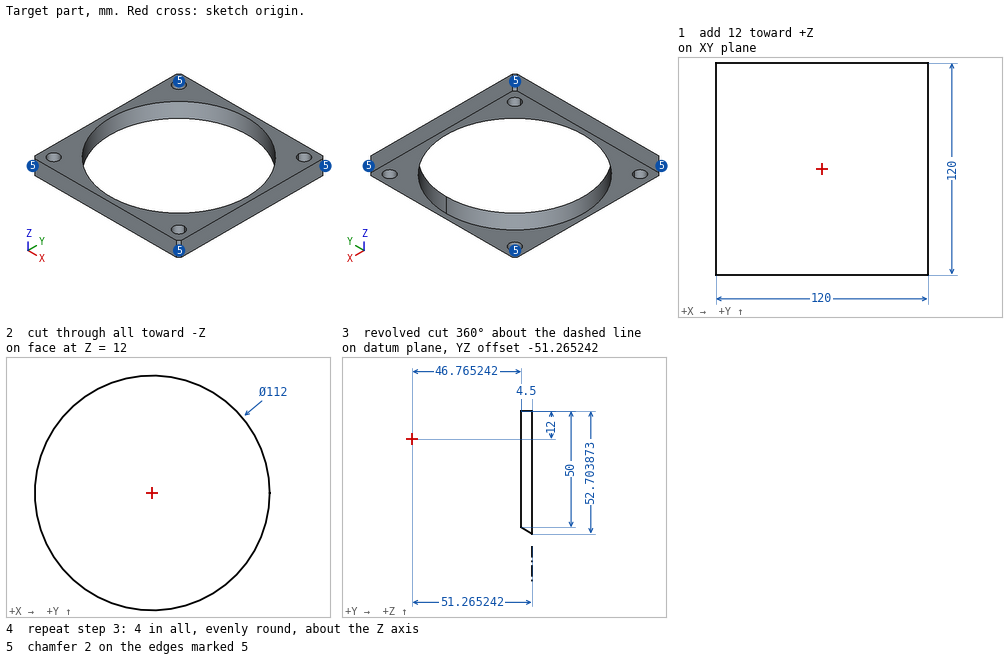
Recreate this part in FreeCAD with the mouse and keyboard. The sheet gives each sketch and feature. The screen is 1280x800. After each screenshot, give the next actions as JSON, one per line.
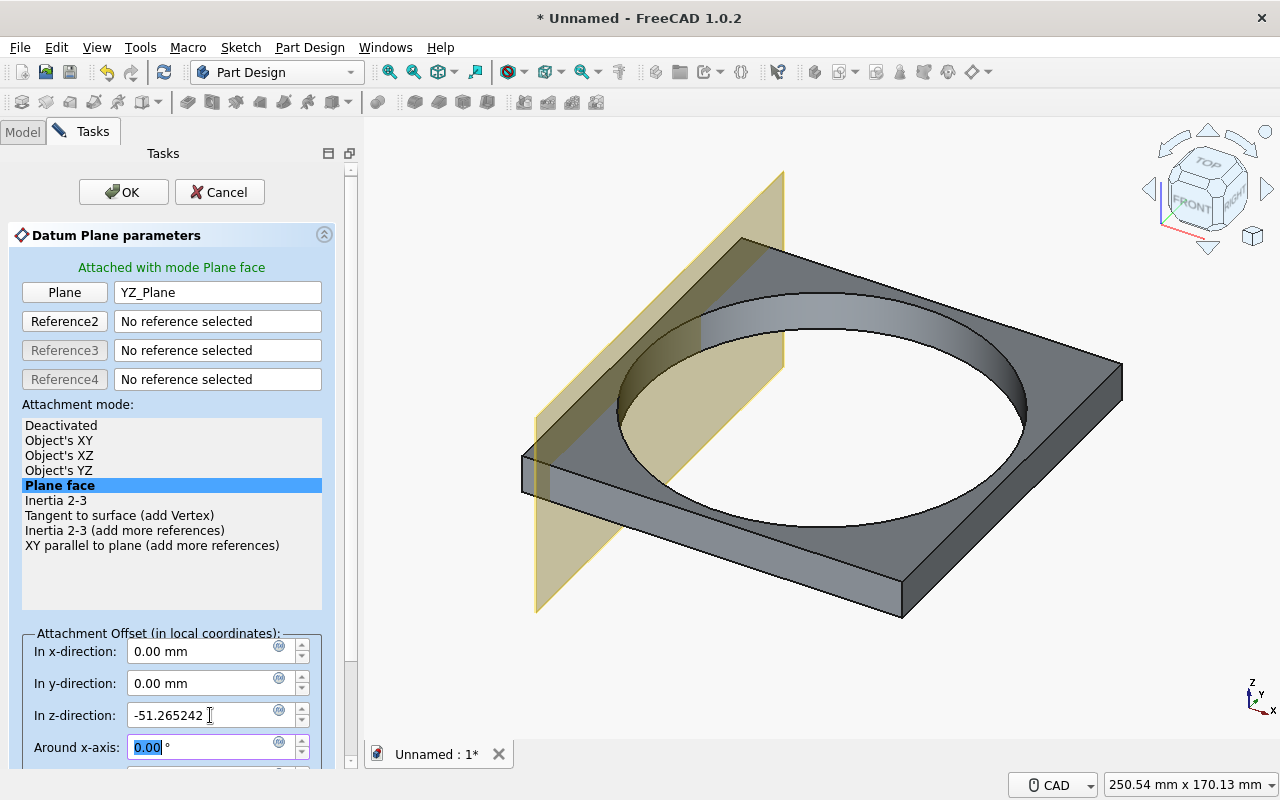
{"action": "left_click", "coordinate": [124, 192]}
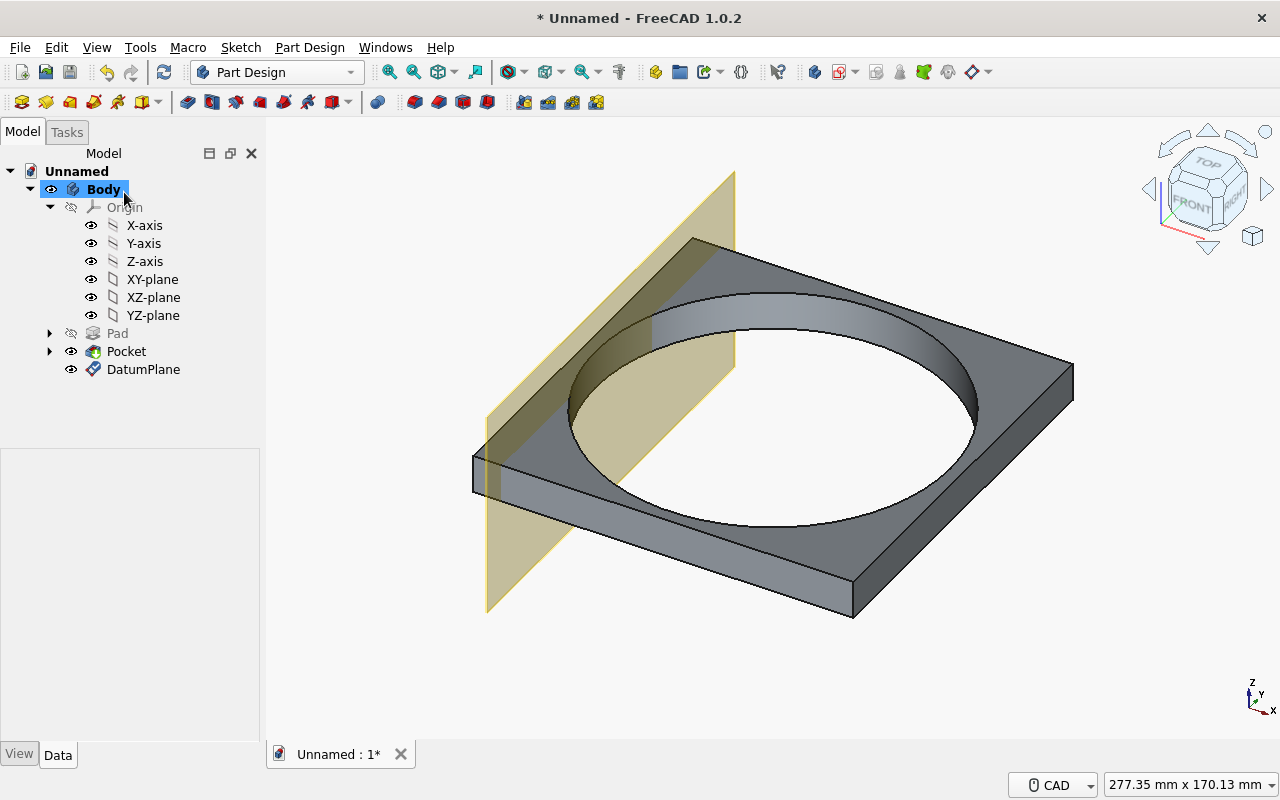
{"action": "left_click", "coordinate": [116, 369]}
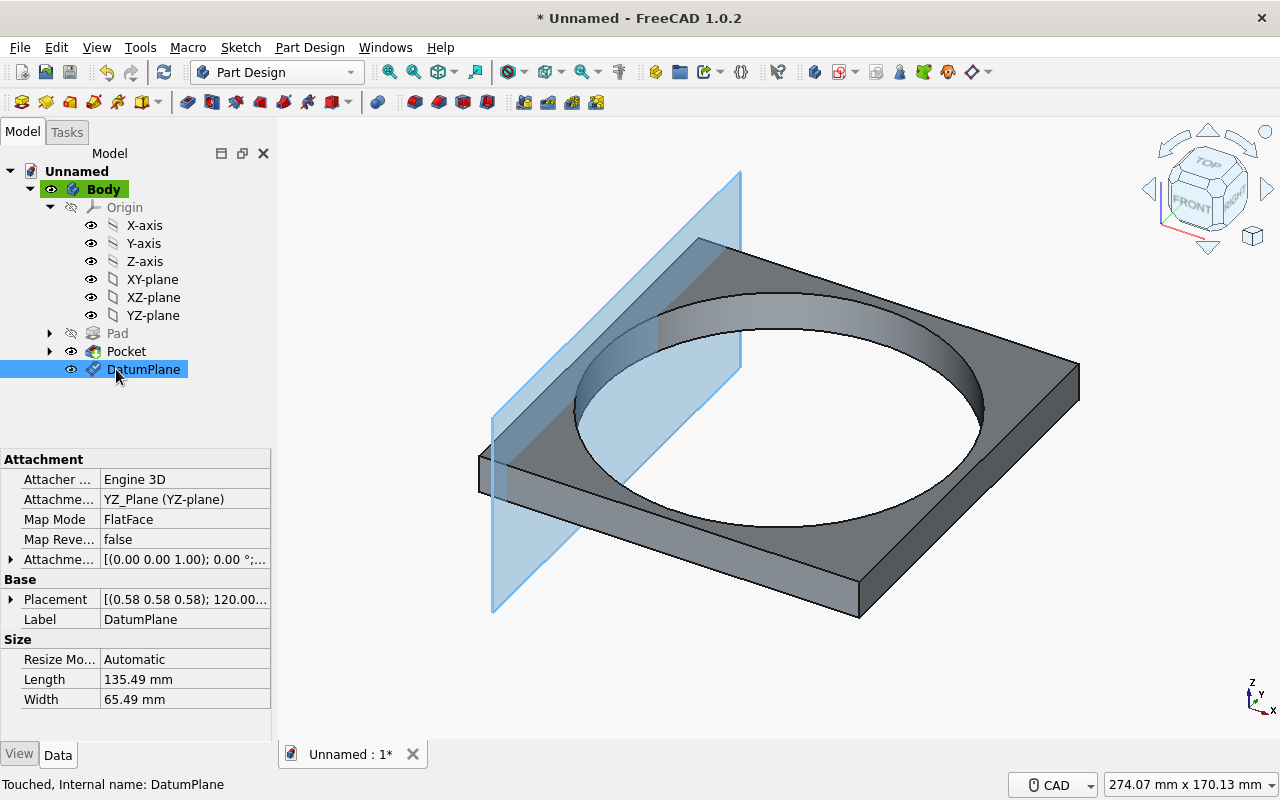
{"action": "left_click", "coordinate": [840, 72]}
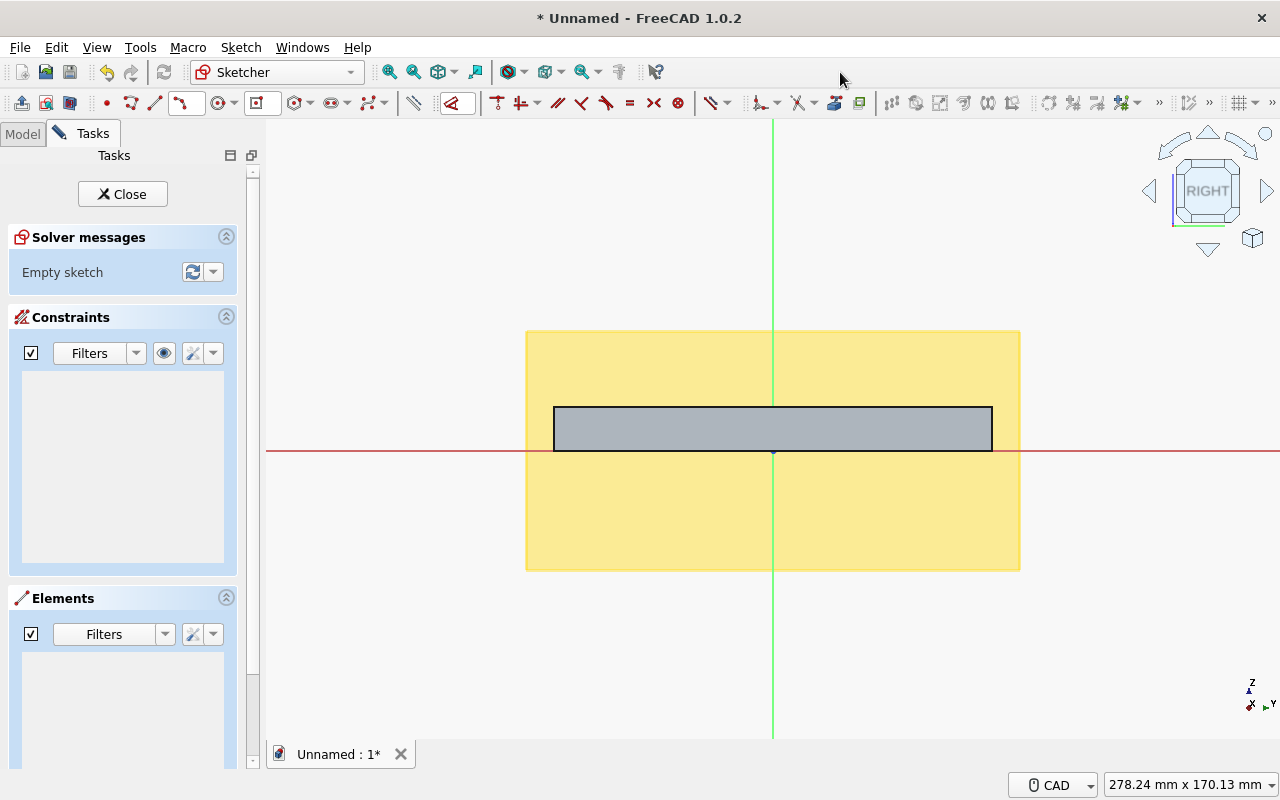
{"action": "key", "text": "q s"}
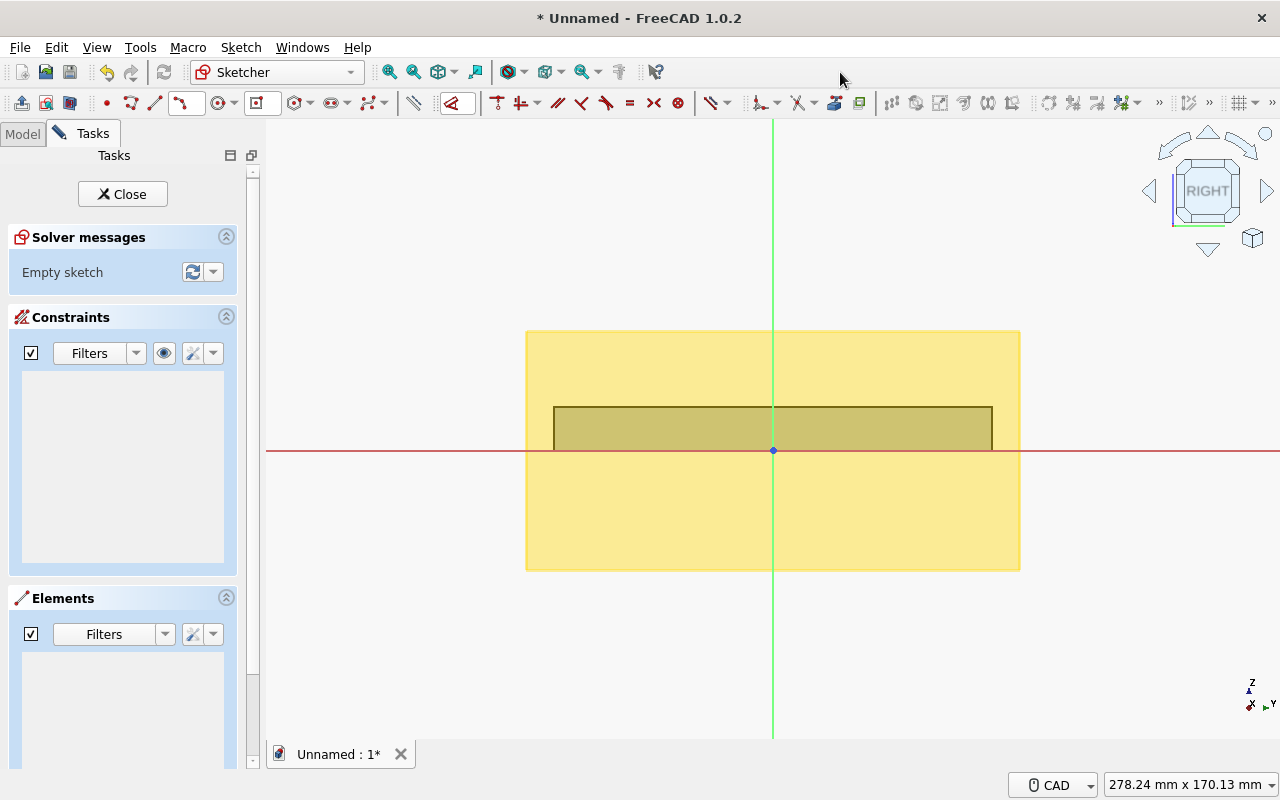
{"action": "scroll", "coordinate": [1115, 711], "scroll_direction": "up", "scroll_amount": 2}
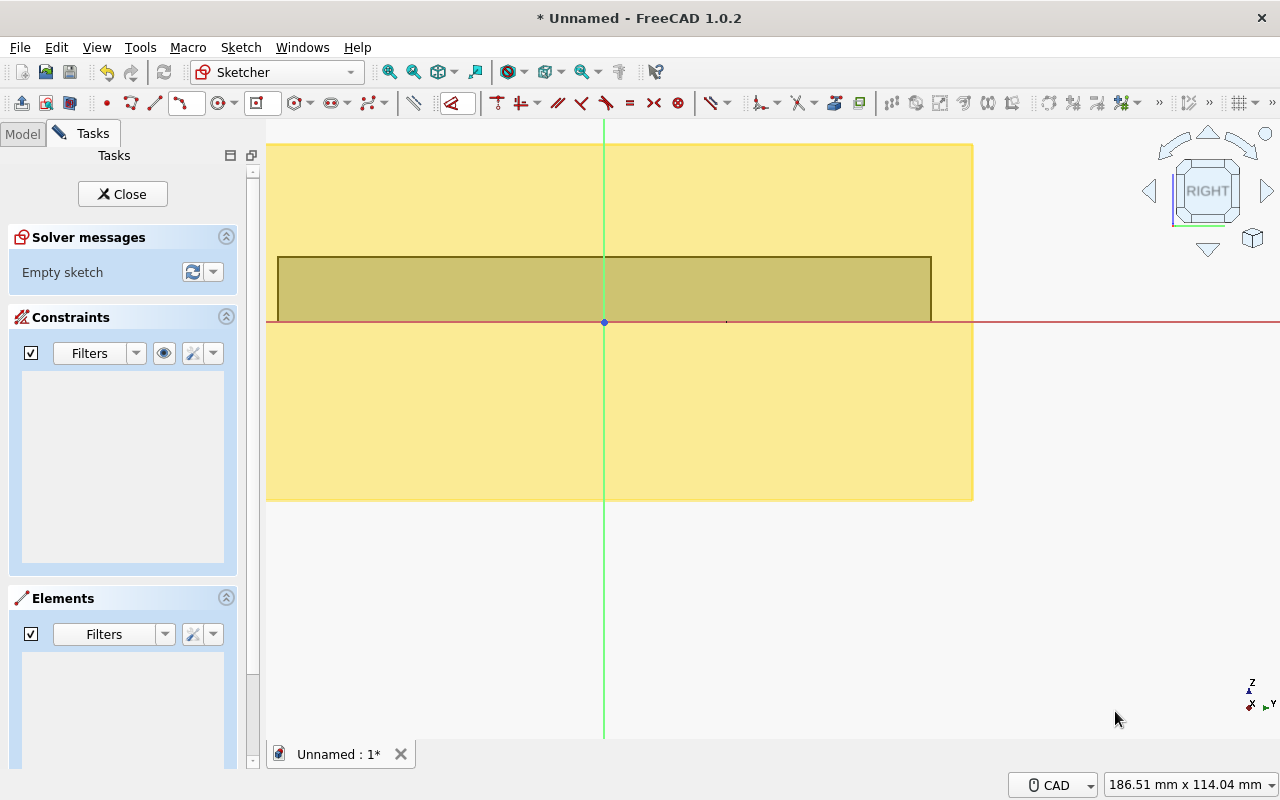
{"action": "left_click", "coordinate": [132, 104]}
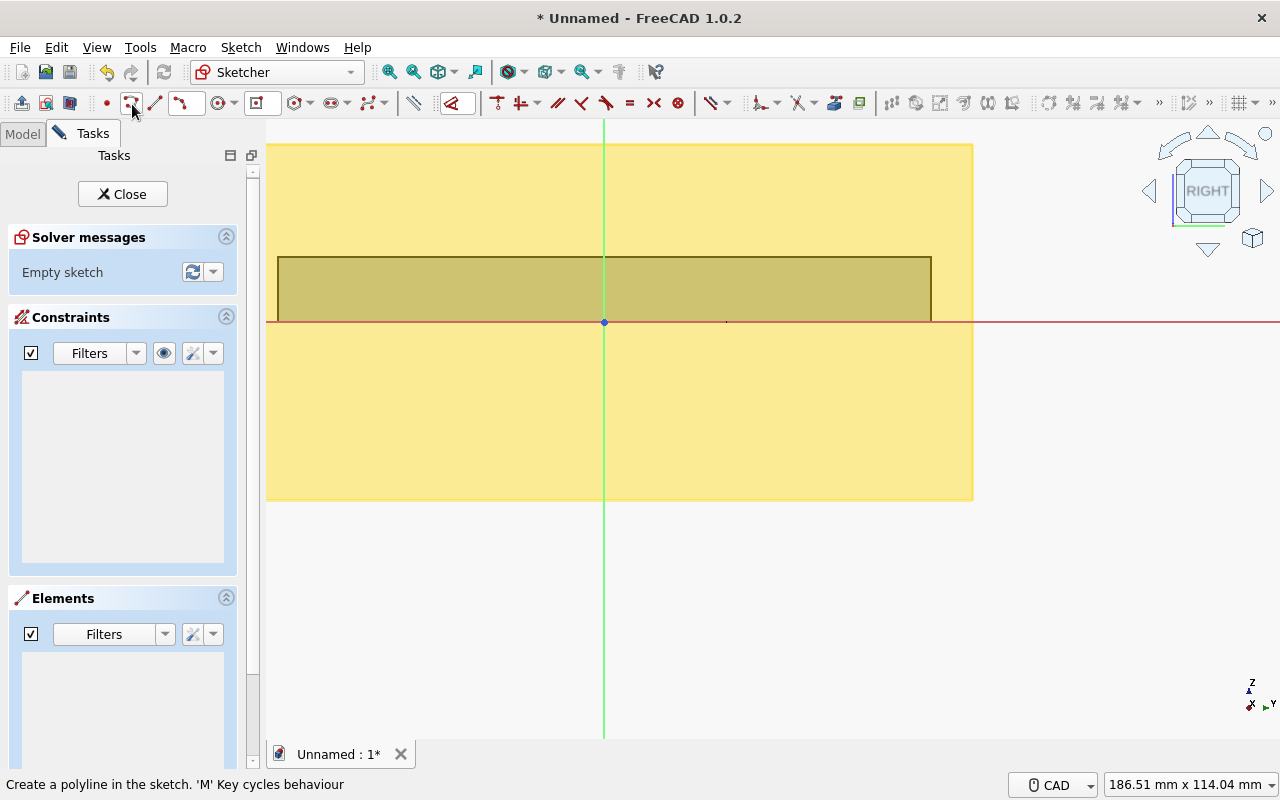
{"action": "left_click", "coordinate": [859, 257]}
{"action": "left_click", "coordinate": [859, 529]}
{"action": "left_click", "coordinate": [883, 544]}
{"action": "left_click", "coordinate": [883, 257]}
{"action": "left_click", "coordinate": [859, 258]}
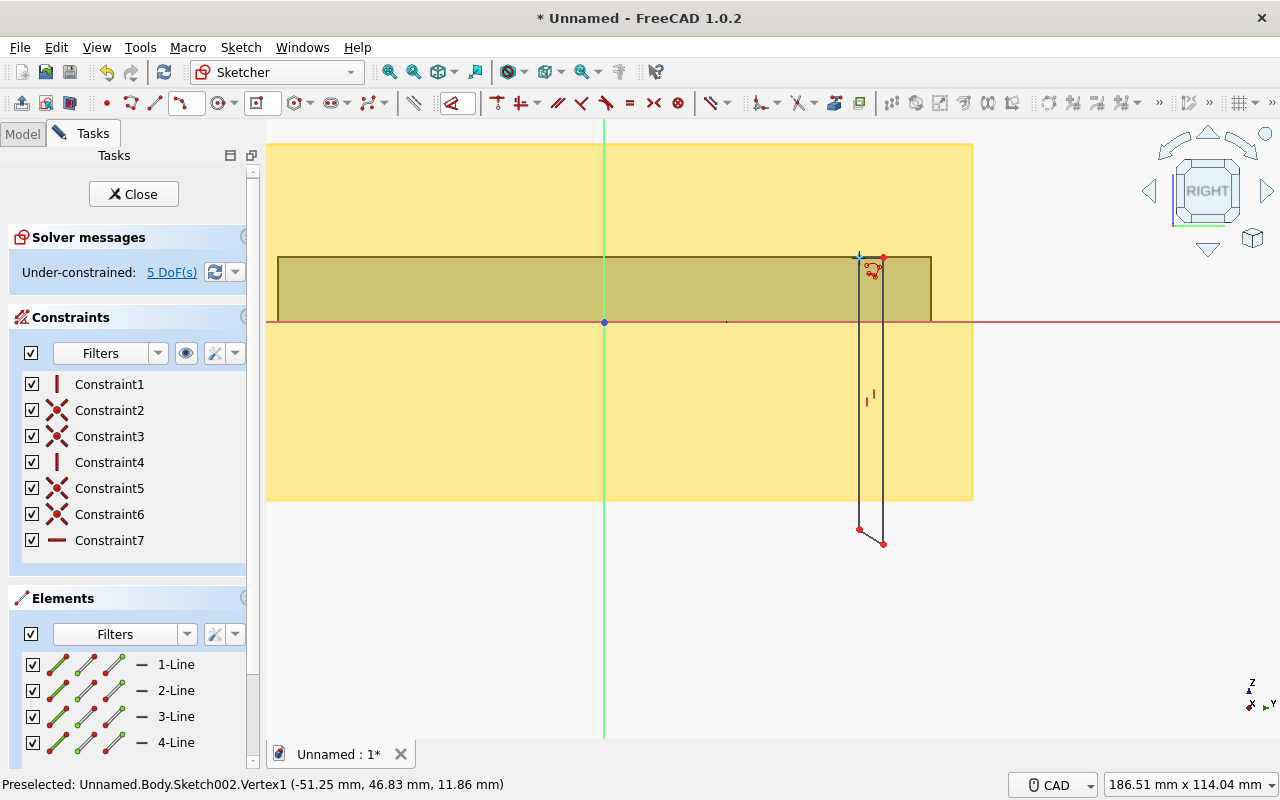
{"action": "left_click", "coordinate": [156, 104]}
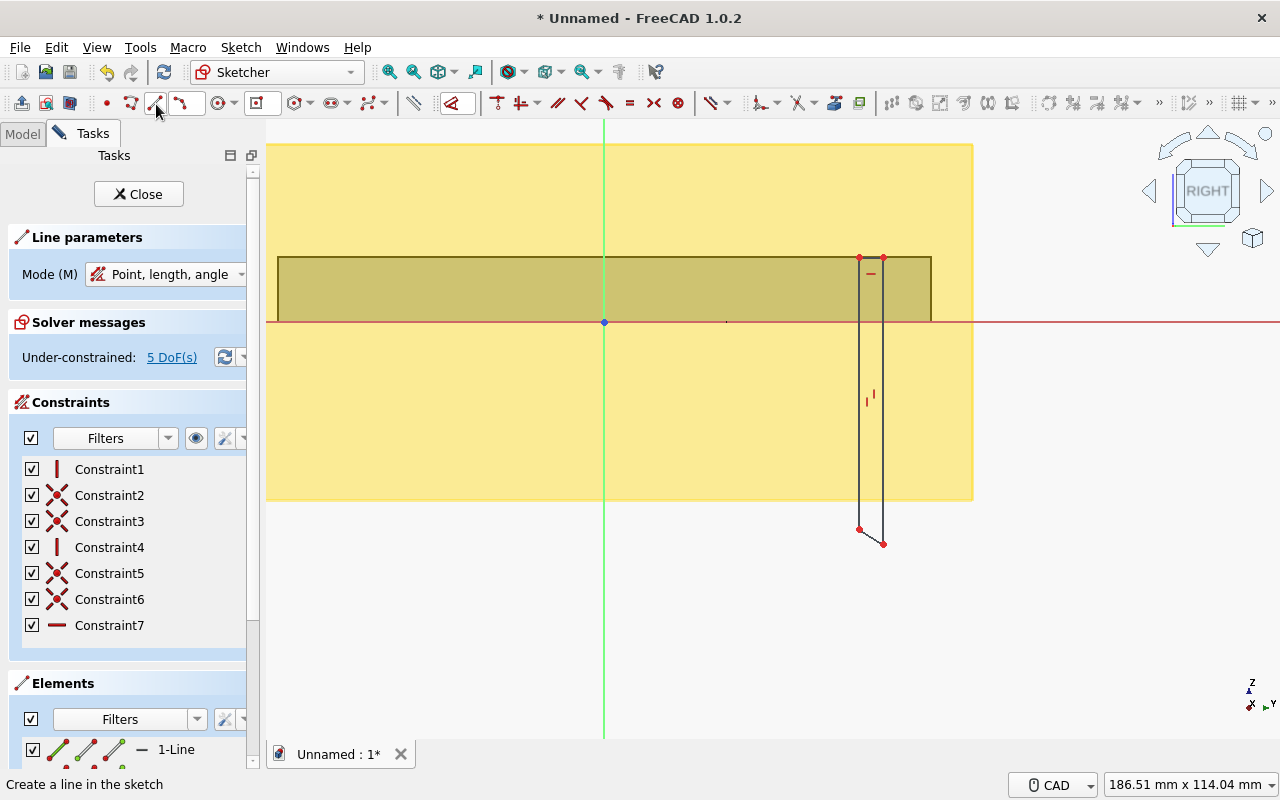
{"action": "left_click", "coordinate": [883, 572]}
{"action": "left_click", "coordinate": [883, 658]}
{"action": "key", "text": "Escape"}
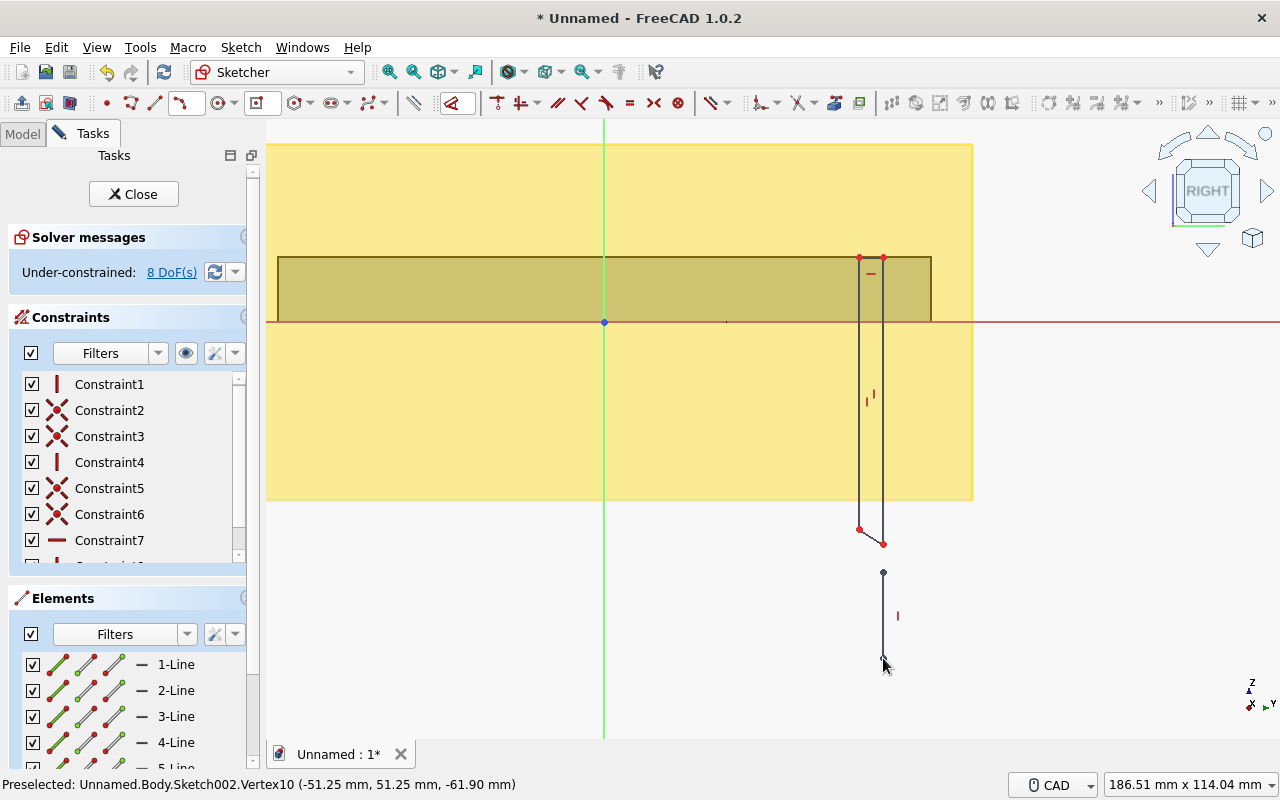
{"action": "left_click", "coordinate": [883, 599]}